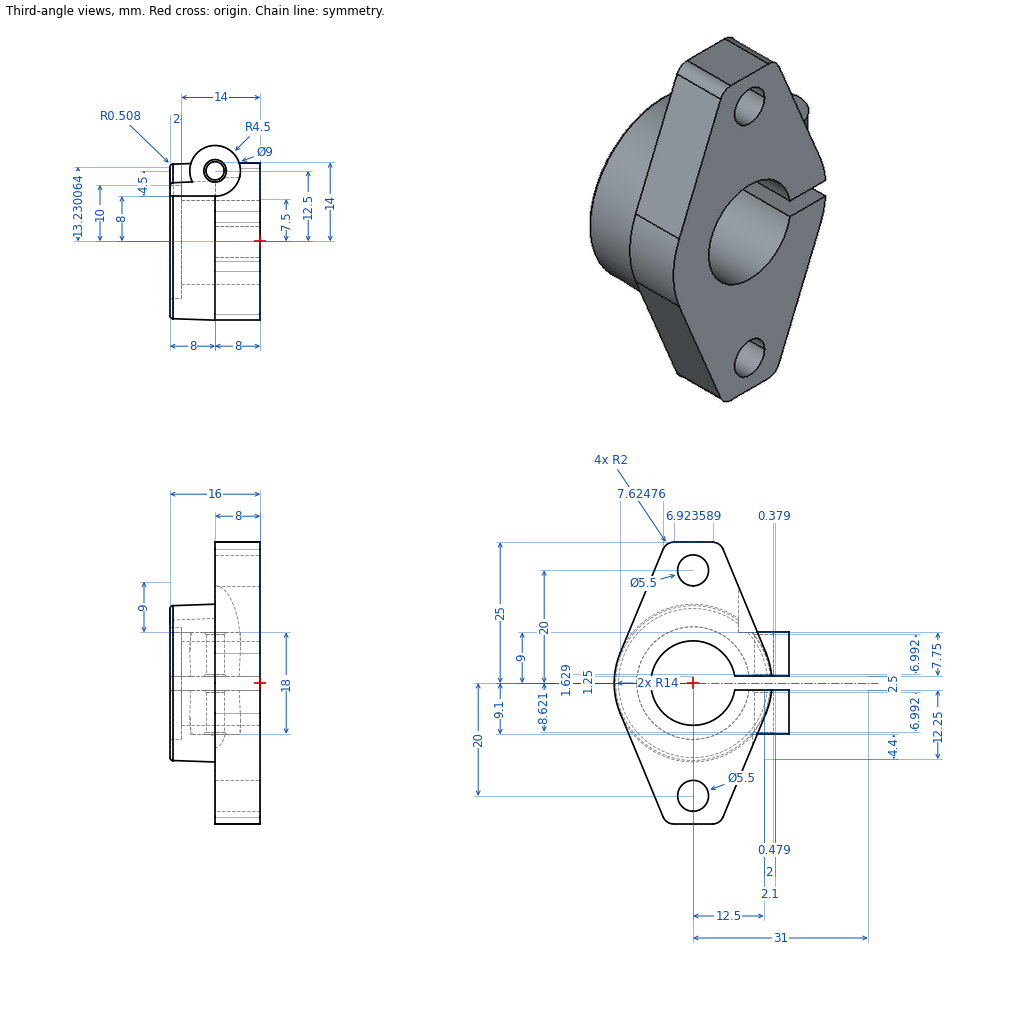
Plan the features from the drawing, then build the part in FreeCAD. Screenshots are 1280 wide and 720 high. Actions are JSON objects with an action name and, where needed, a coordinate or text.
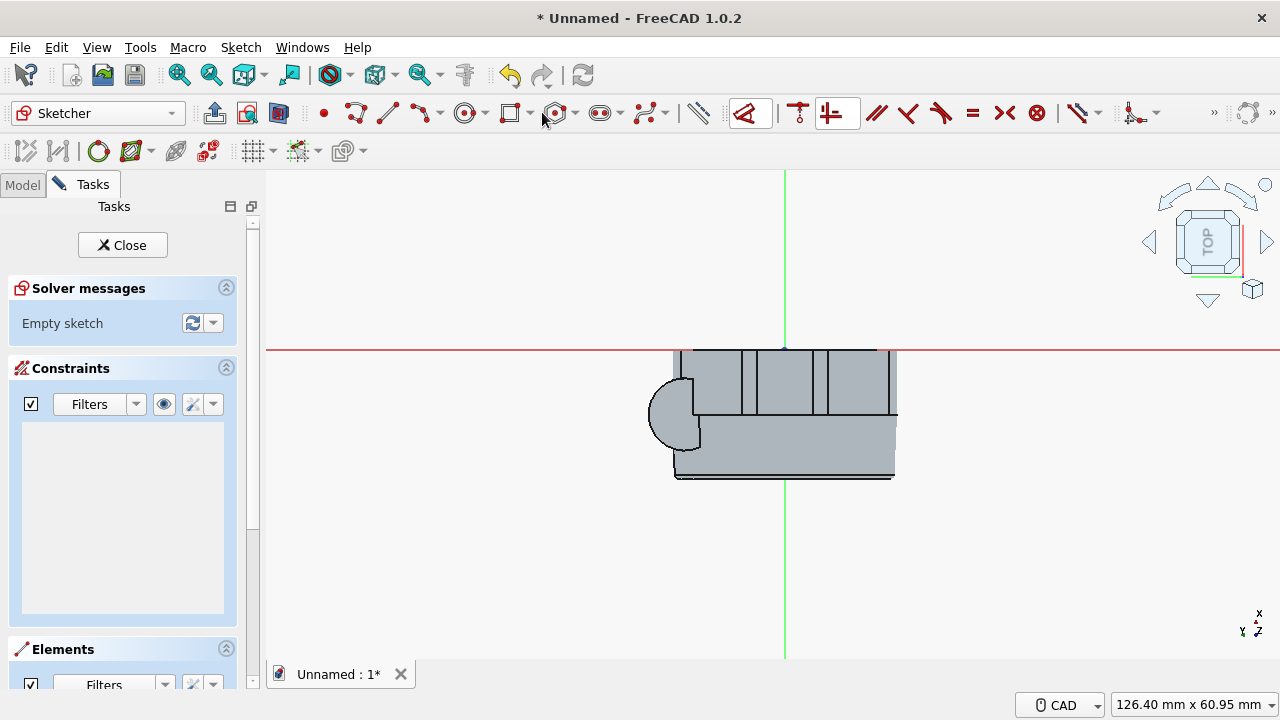
{"action": "left_click", "coordinate": [280, 114]}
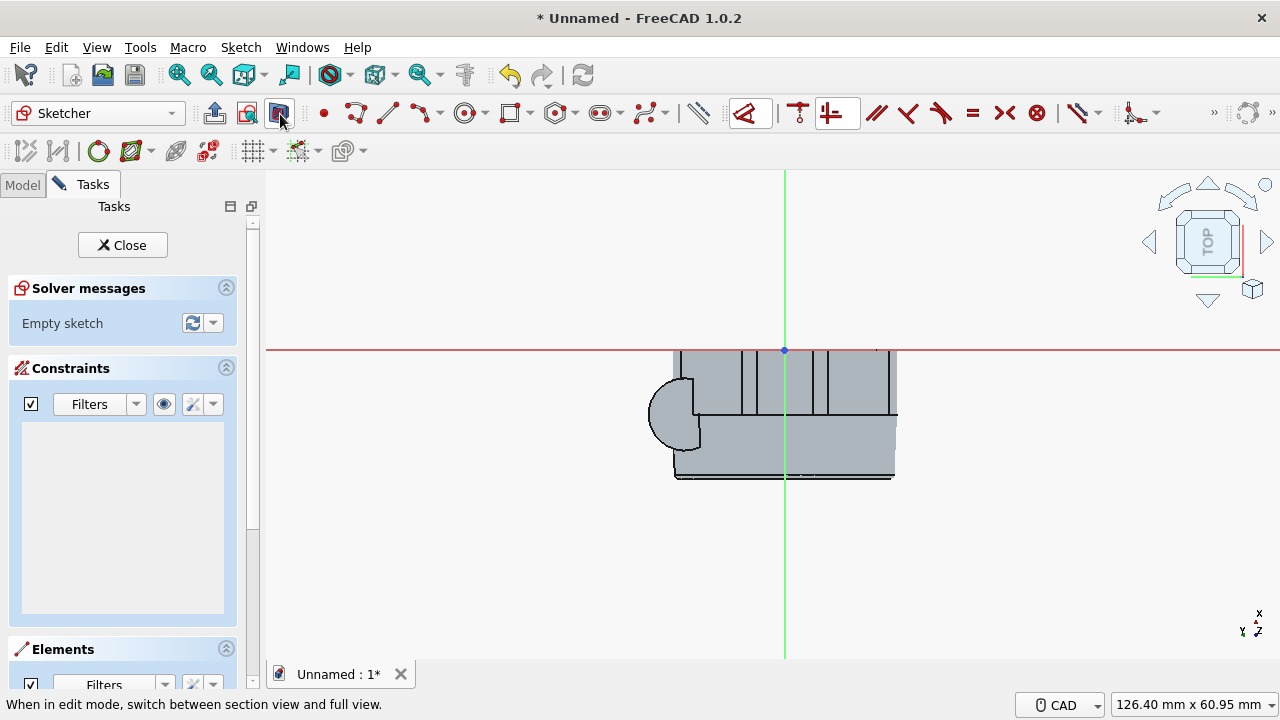
{"action": "scroll", "coordinate": [736, 414], "scroll_direction": "up", "scroll_amount": 4}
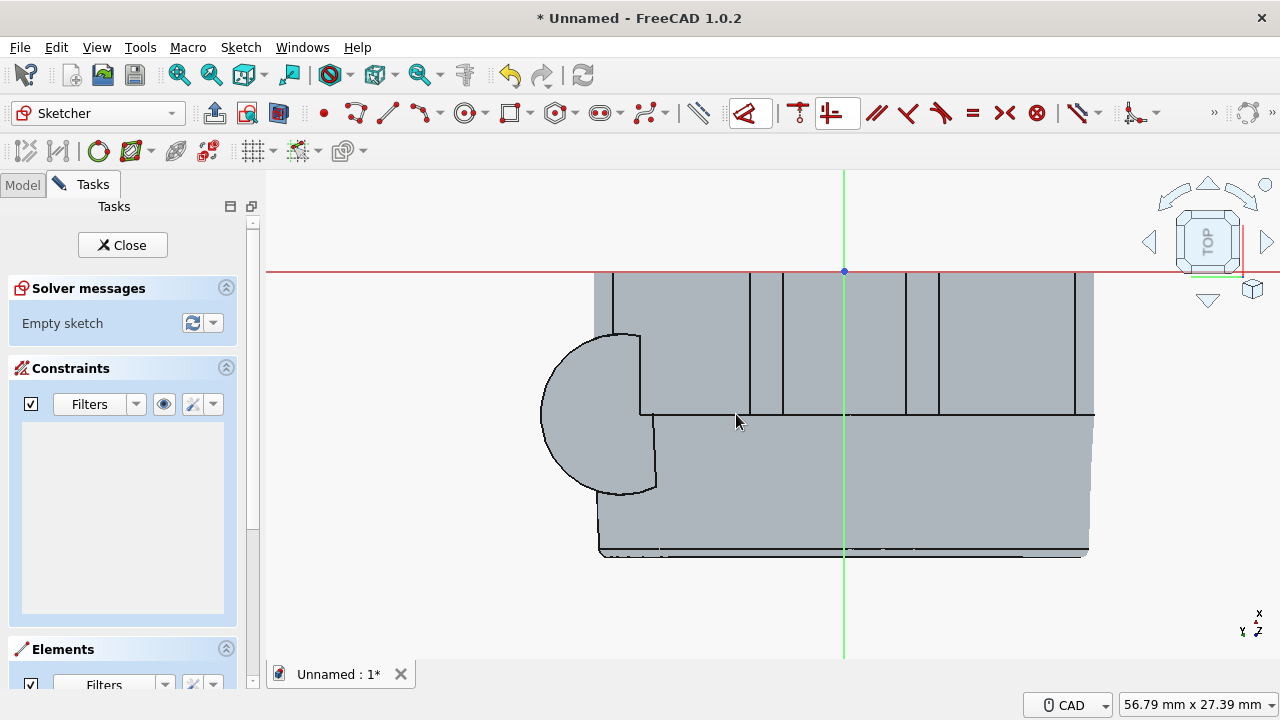
{"action": "key", "text": "g m"}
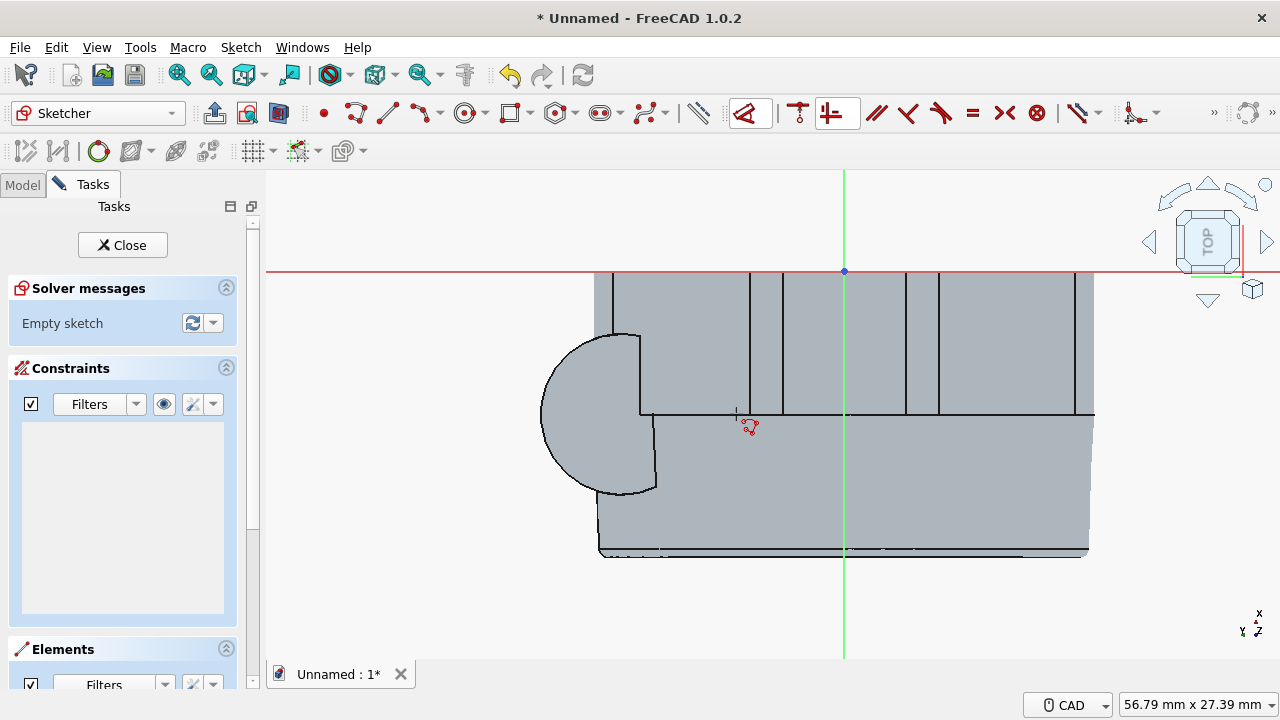
{"action": "left_click", "coordinate": [621, 495]}
{"action": "left_click", "coordinate": [621, 557]}
{"action": "left_click", "coordinate": [702, 557]}
{"action": "left_click", "coordinate": [702, 415]}
{"action": "right_click", "coordinate": [702, 415]}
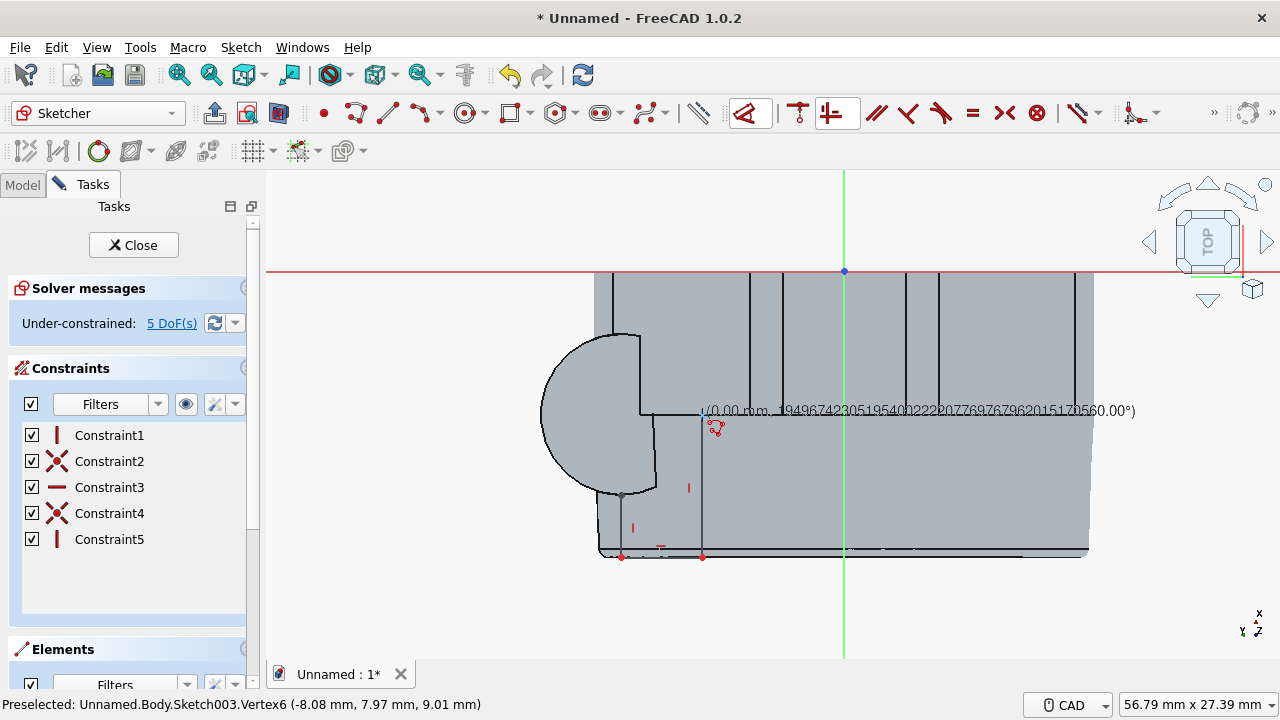
{"action": "left_click", "coordinate": [420, 114]}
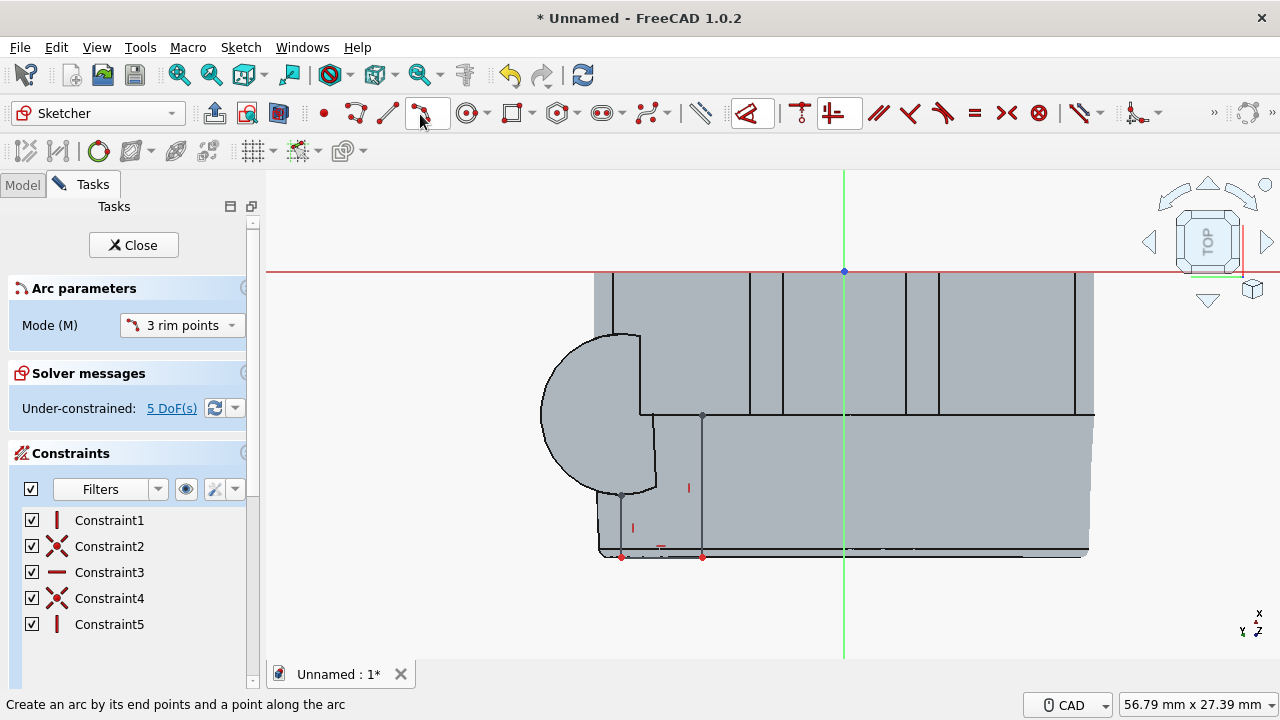
{"action": "left_click", "coordinate": [702, 416]}
{"action": "left_click", "coordinate": [621, 496]}
{"action": "left_click", "coordinate": [564, 358]}
{"action": "key", "text": "Escape"}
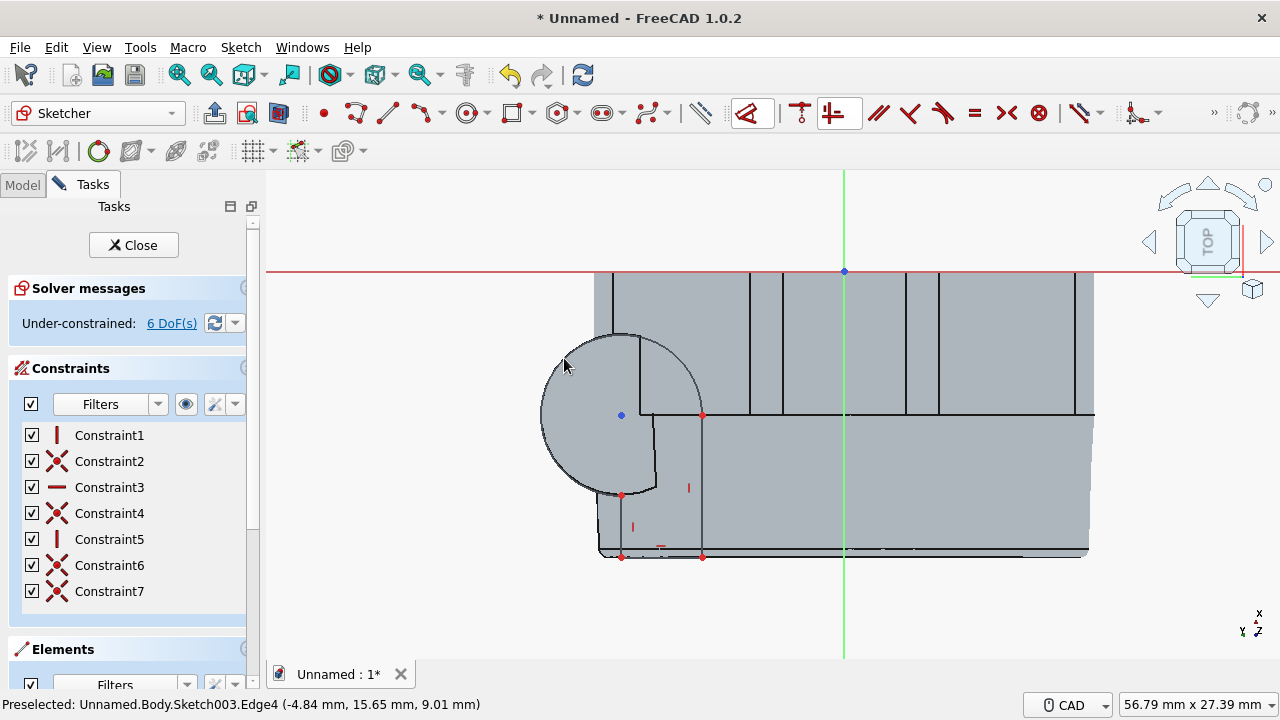
{"action": "left_click", "coordinate": [702, 515]}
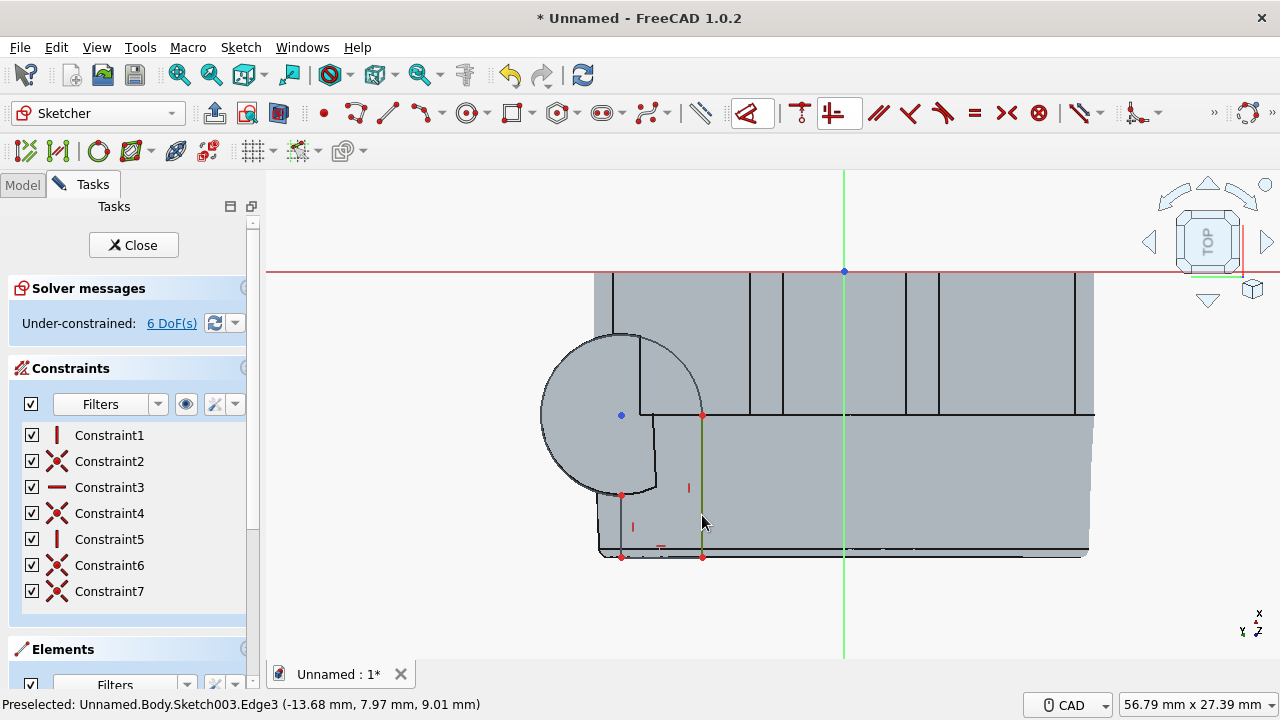
{"action": "left_click", "coordinate": [635, 336]}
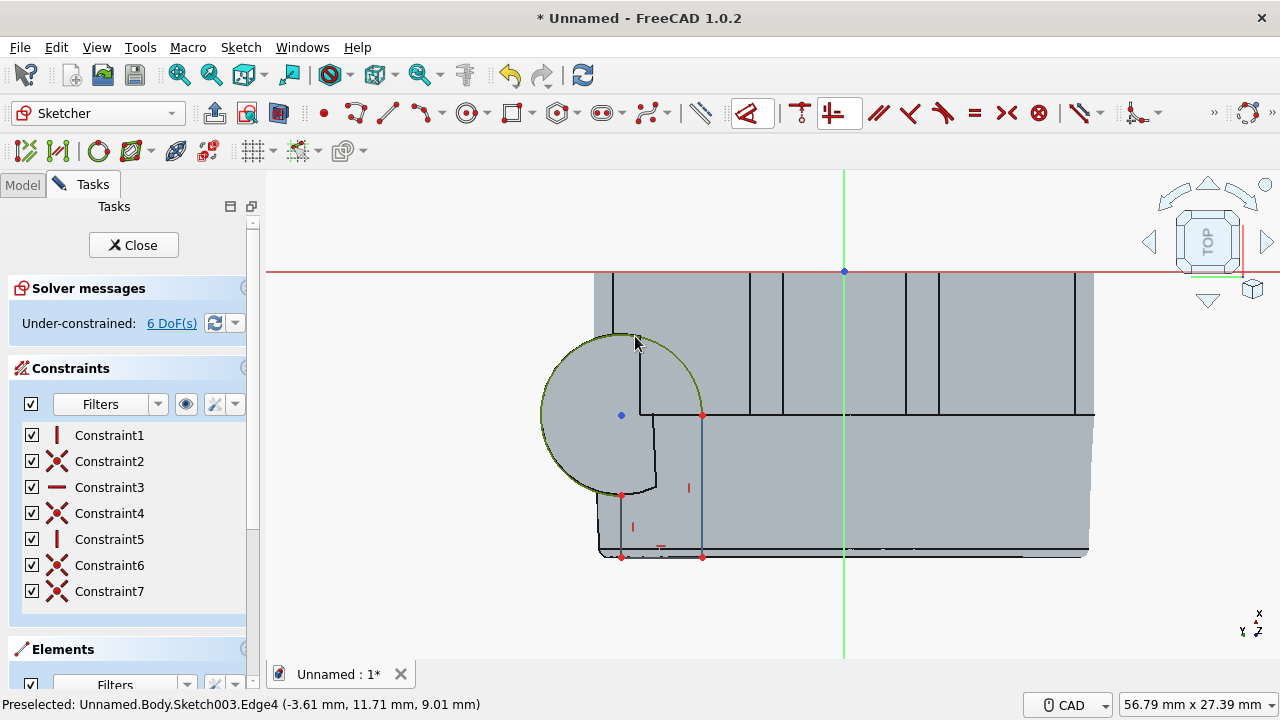
{"action": "left_click", "coordinate": [944, 114]}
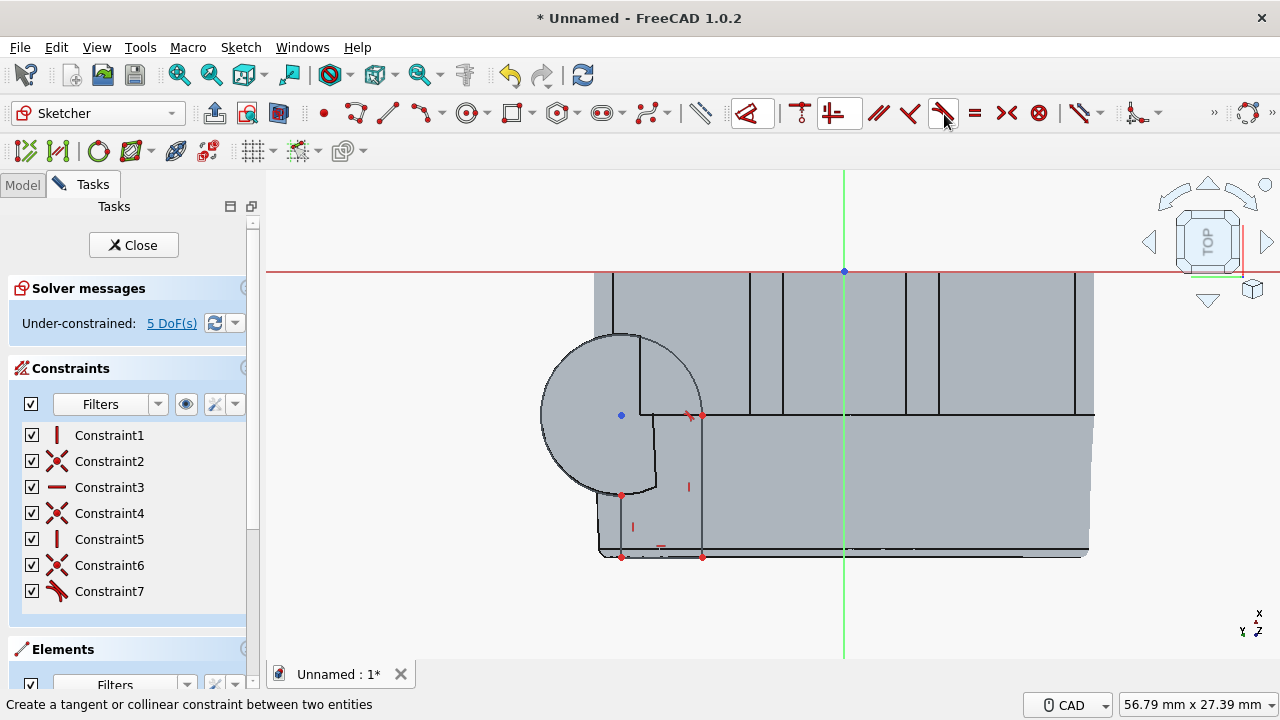
{"action": "left_click", "coordinate": [634, 336]}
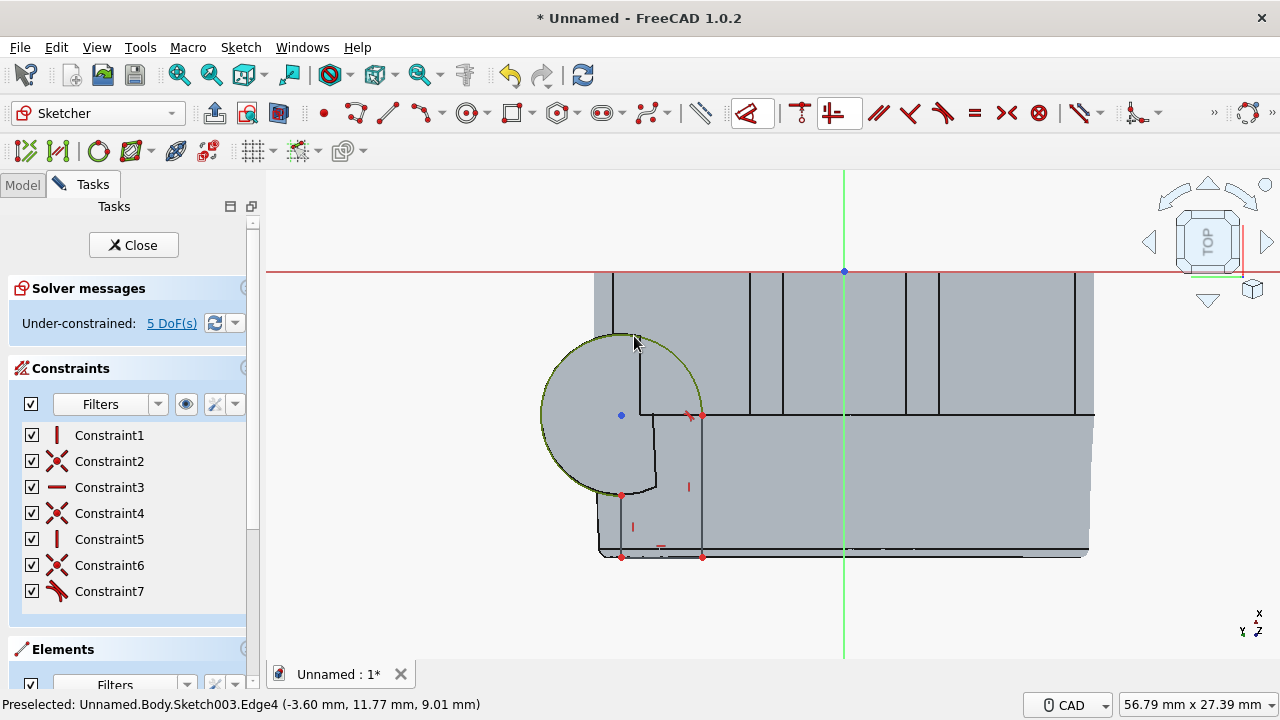
{"action": "key", "text": "k r"}